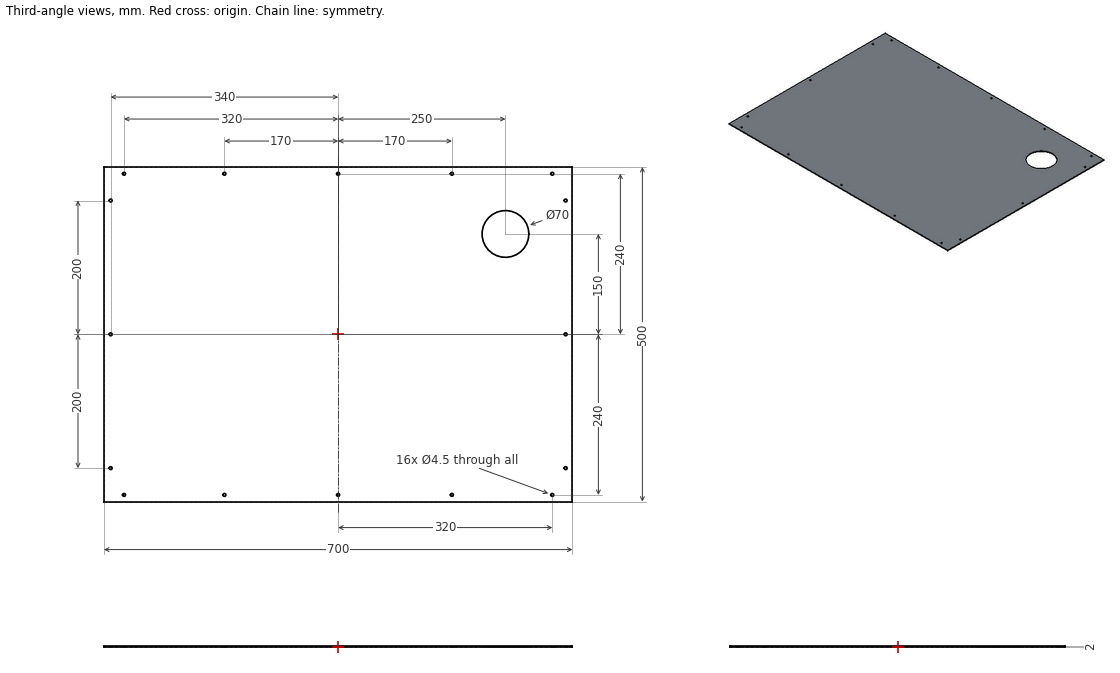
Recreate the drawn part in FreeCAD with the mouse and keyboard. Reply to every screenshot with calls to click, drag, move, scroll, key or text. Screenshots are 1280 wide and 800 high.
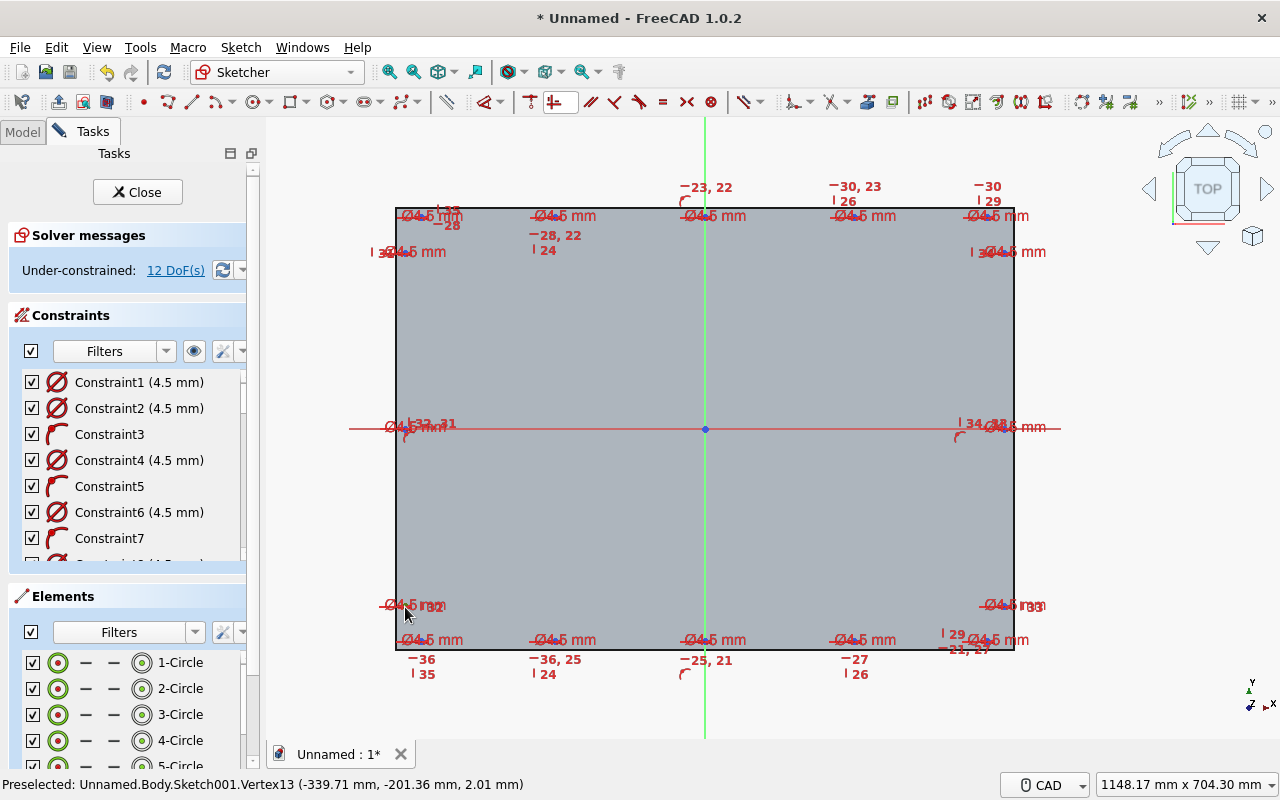
click(1005, 607)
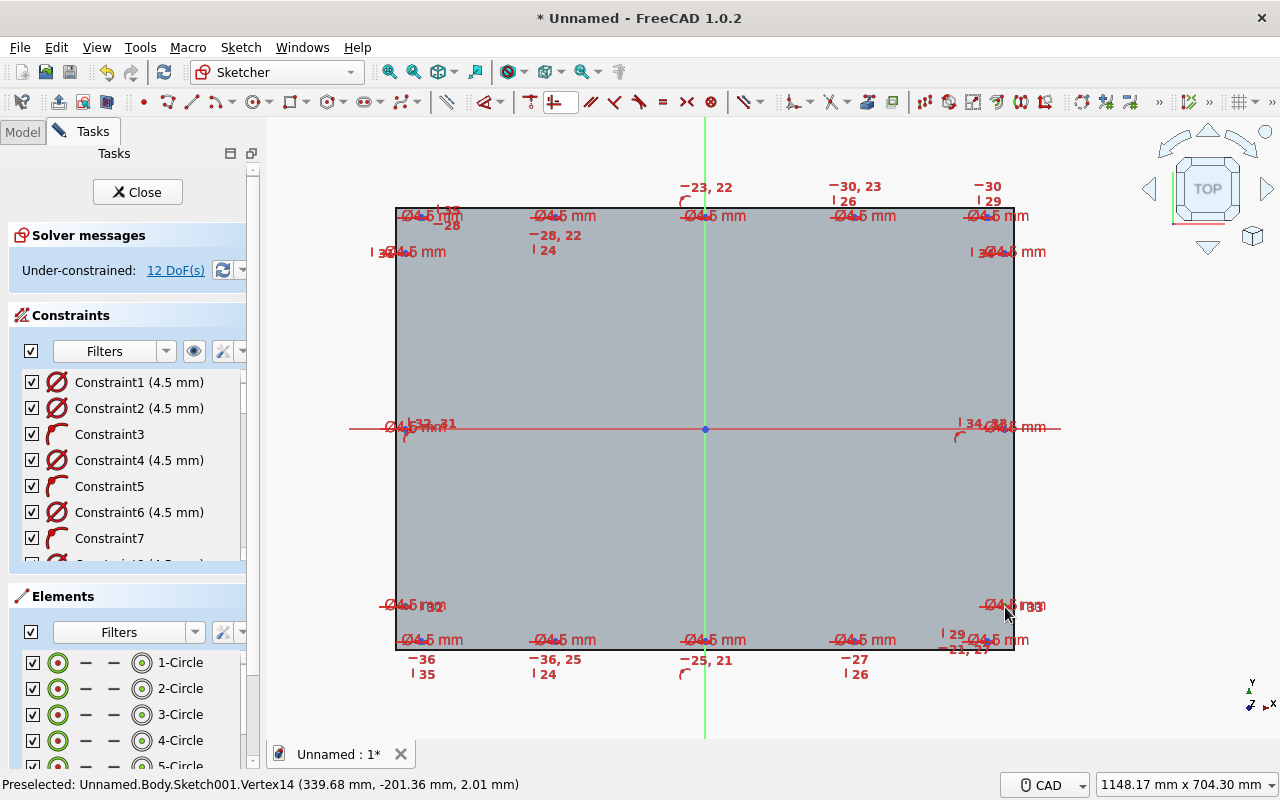
click(705, 590)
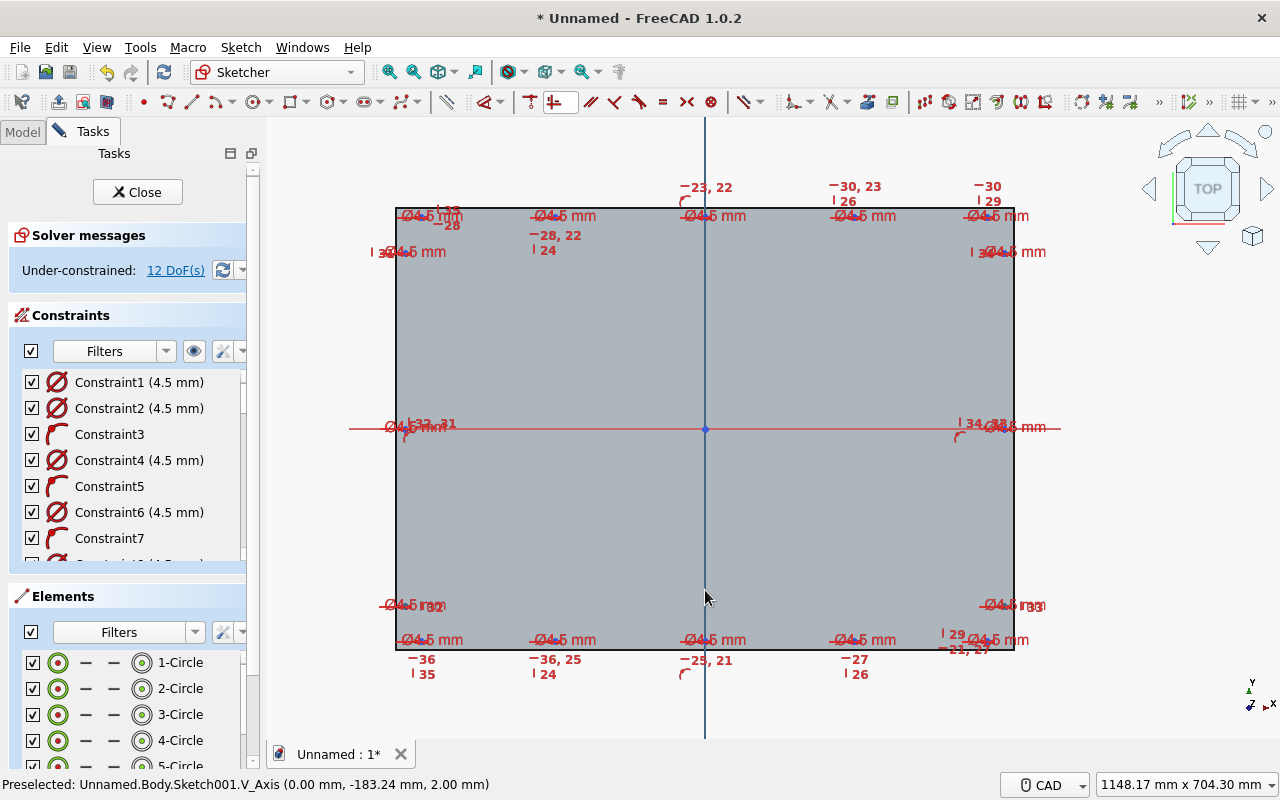
key(s)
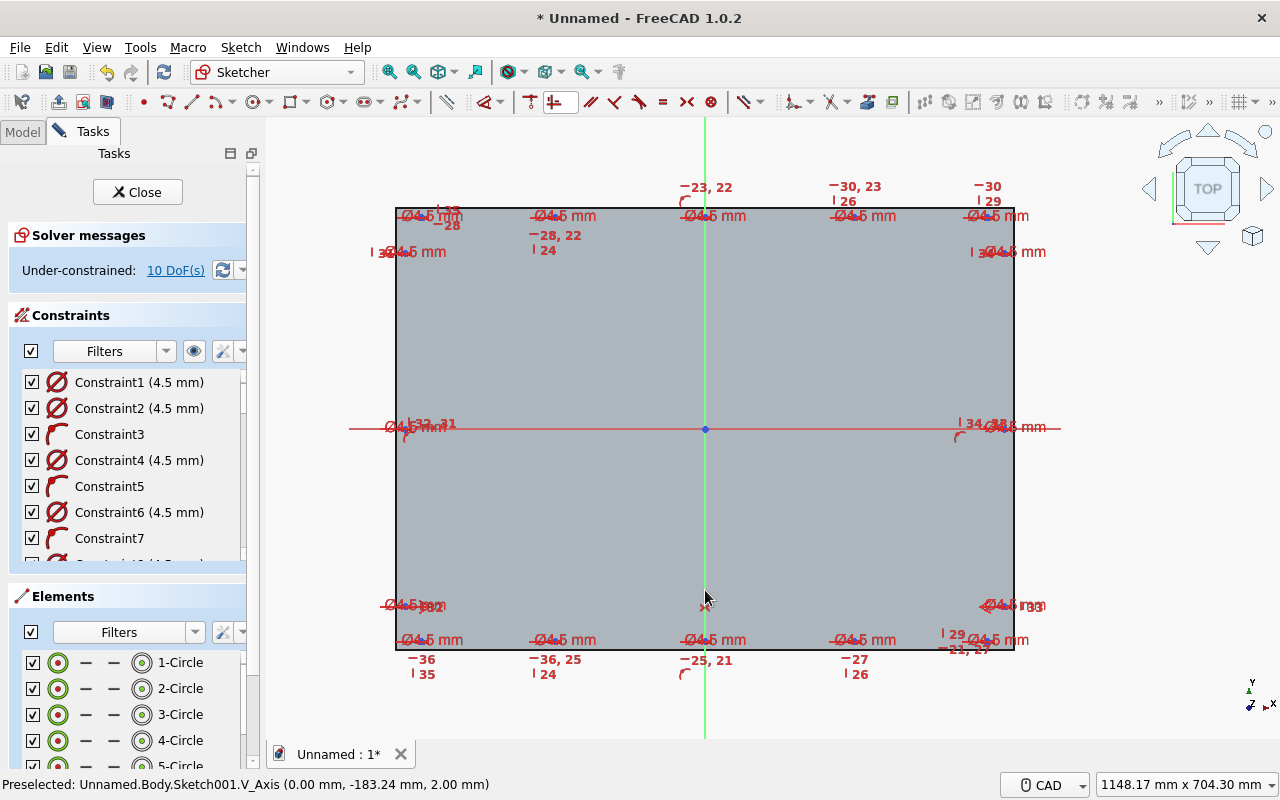
click(484, 102)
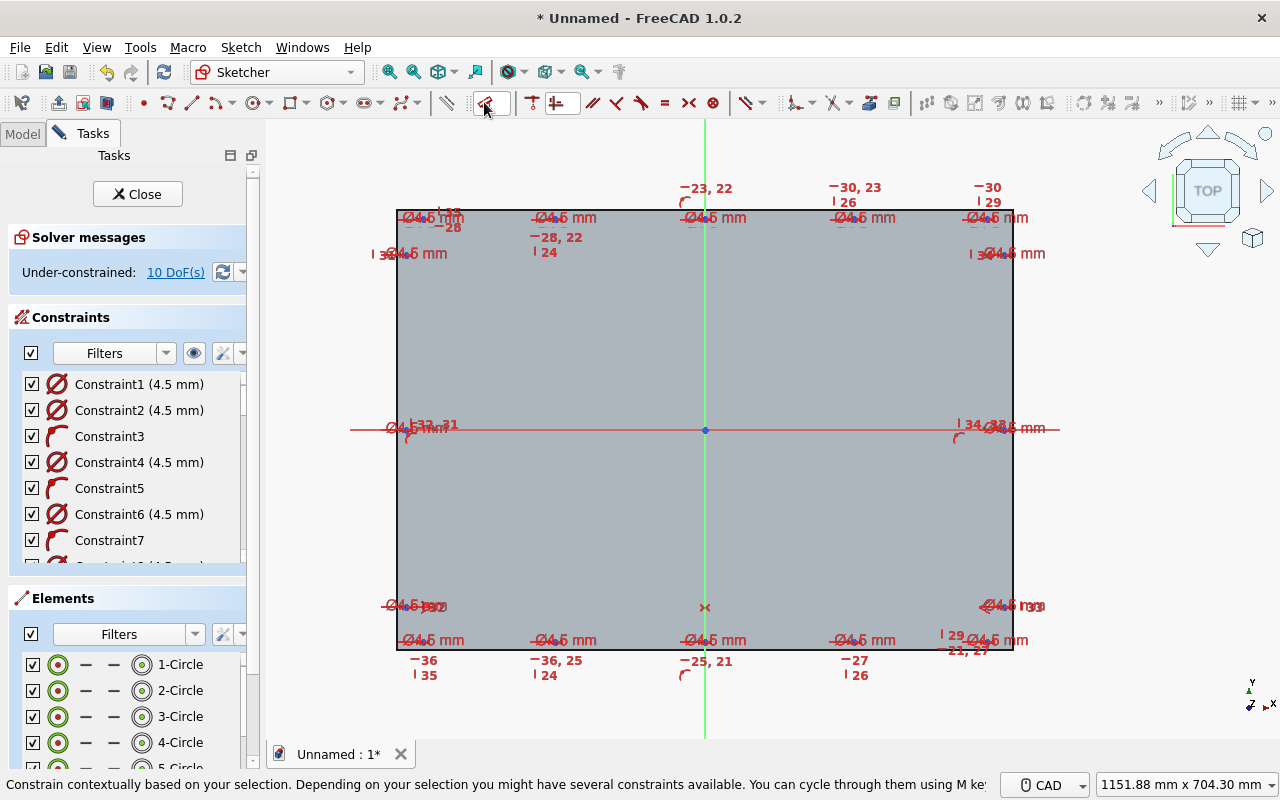
click(987, 642)
click(846, 676)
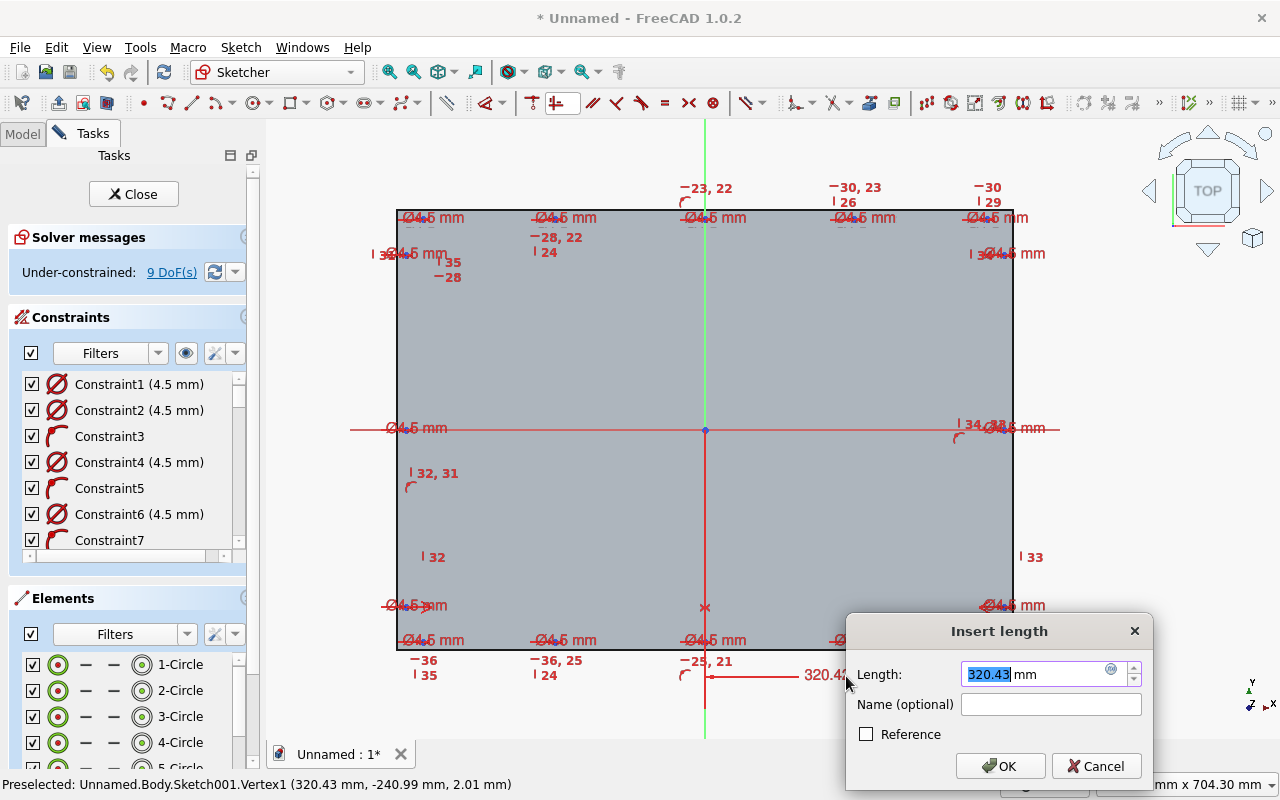
text(320)
key(Return)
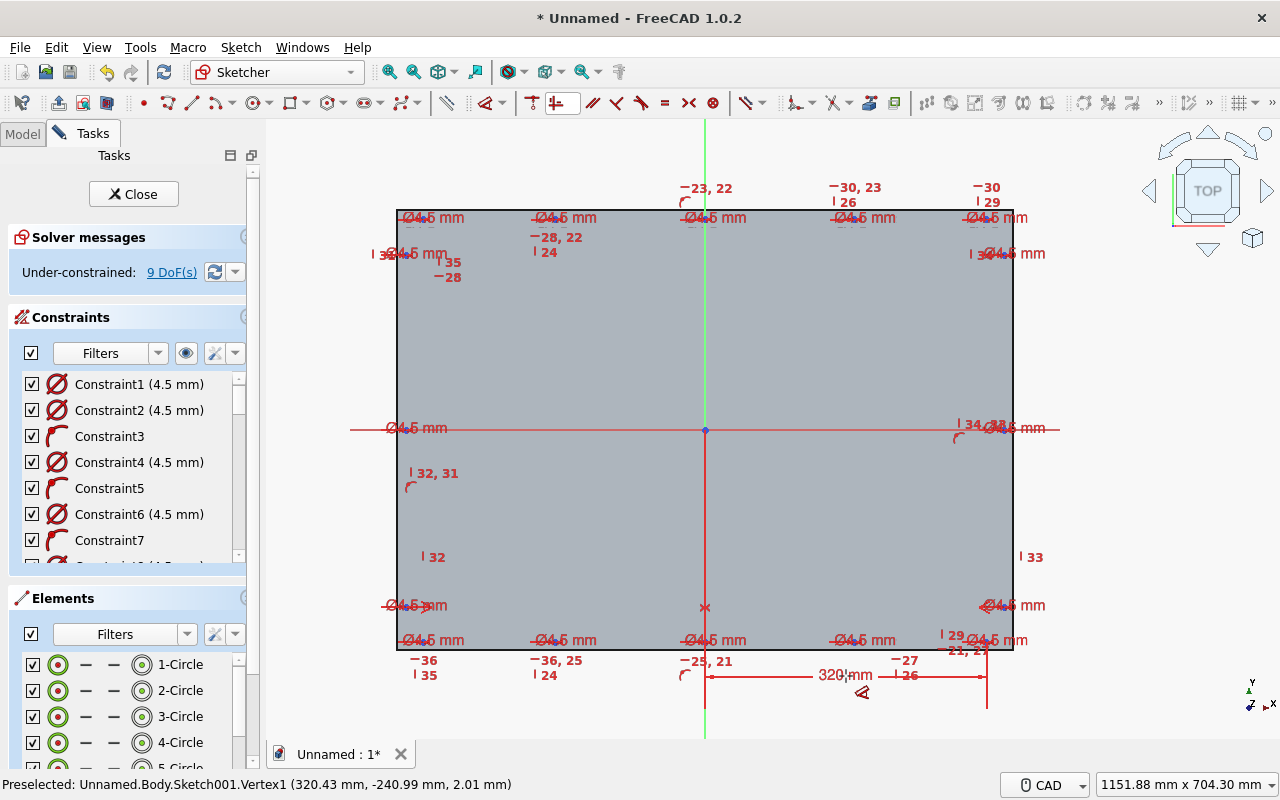
click(987, 642)
click(1021, 536)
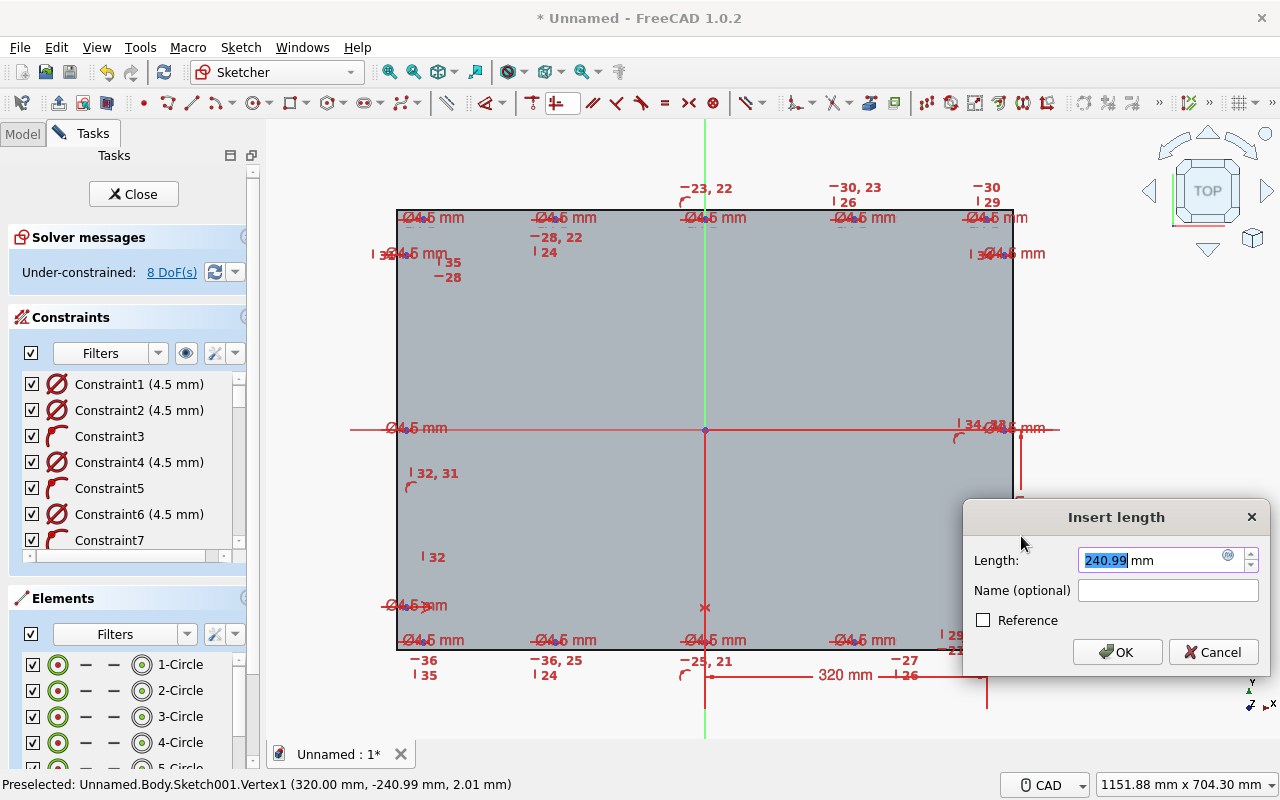
text(240)
key(Return)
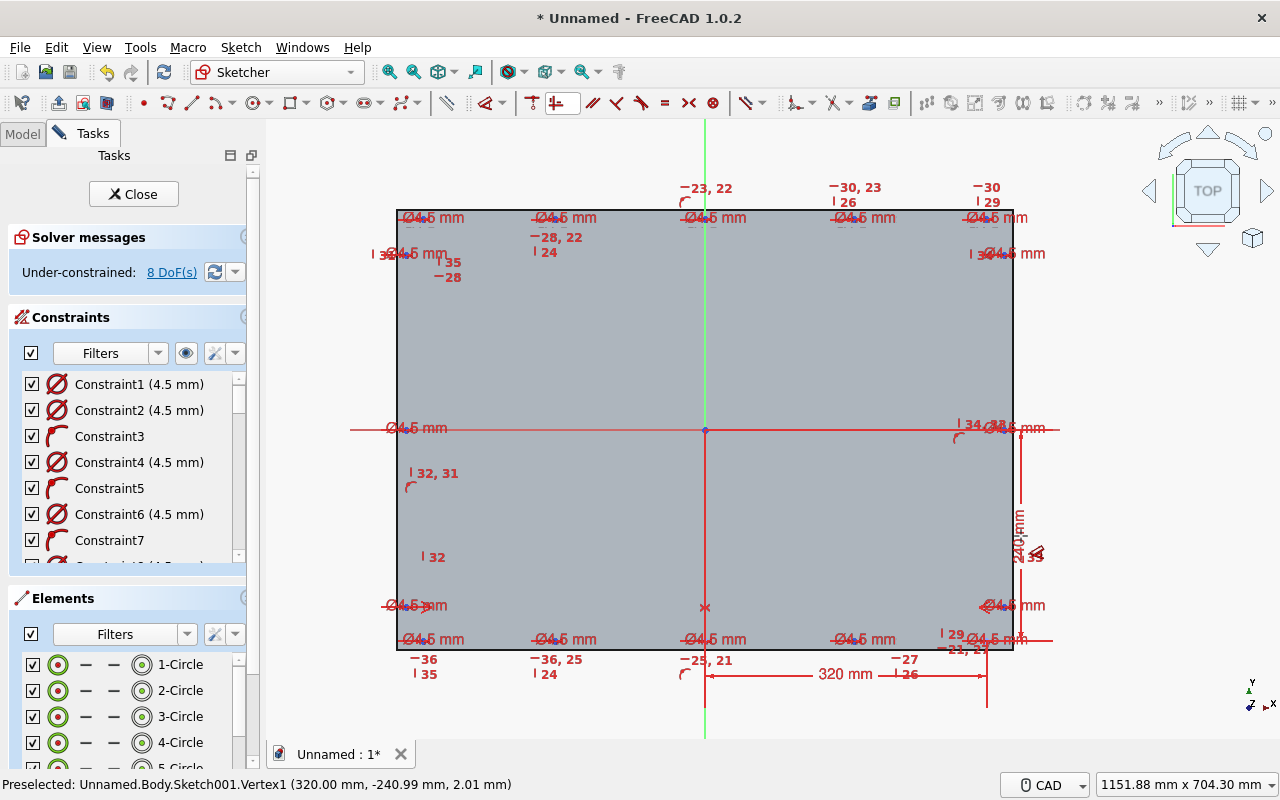
click(406, 430)
click(556, 464)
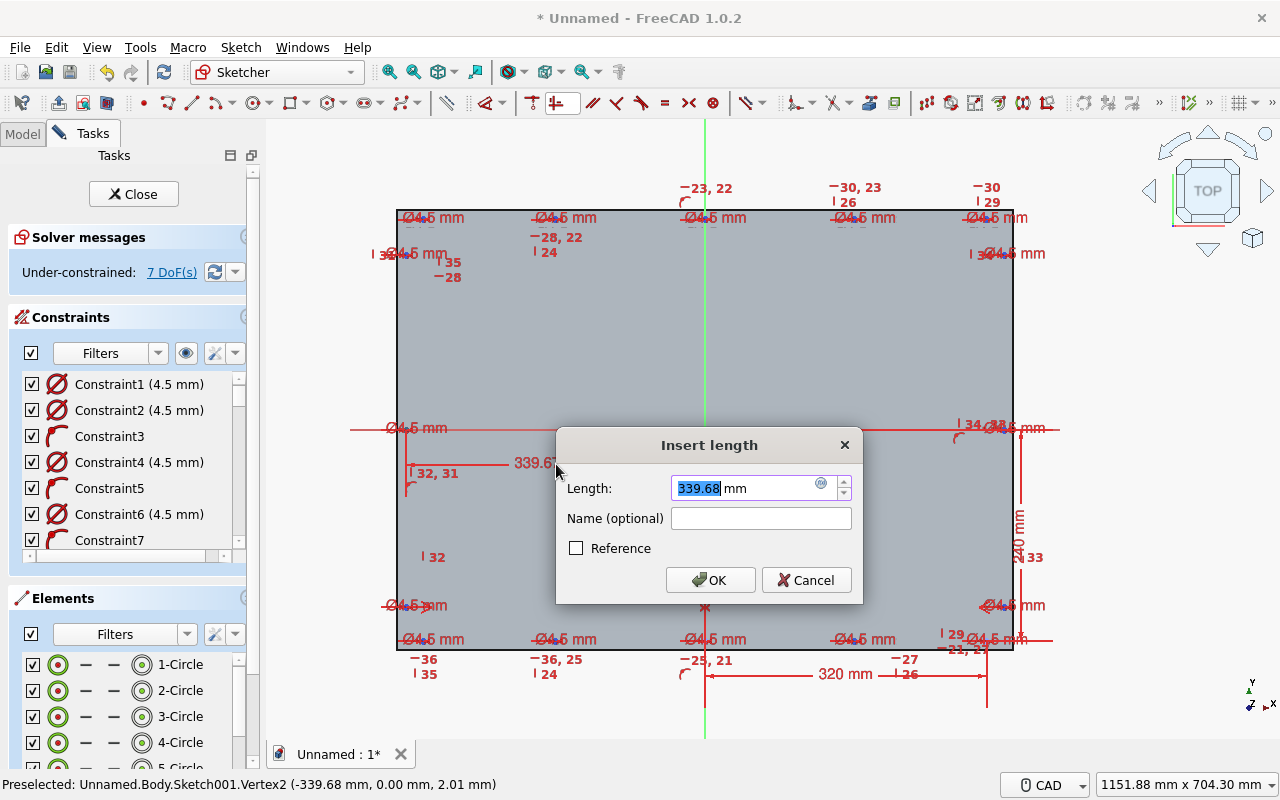
text(340)
key(Return)